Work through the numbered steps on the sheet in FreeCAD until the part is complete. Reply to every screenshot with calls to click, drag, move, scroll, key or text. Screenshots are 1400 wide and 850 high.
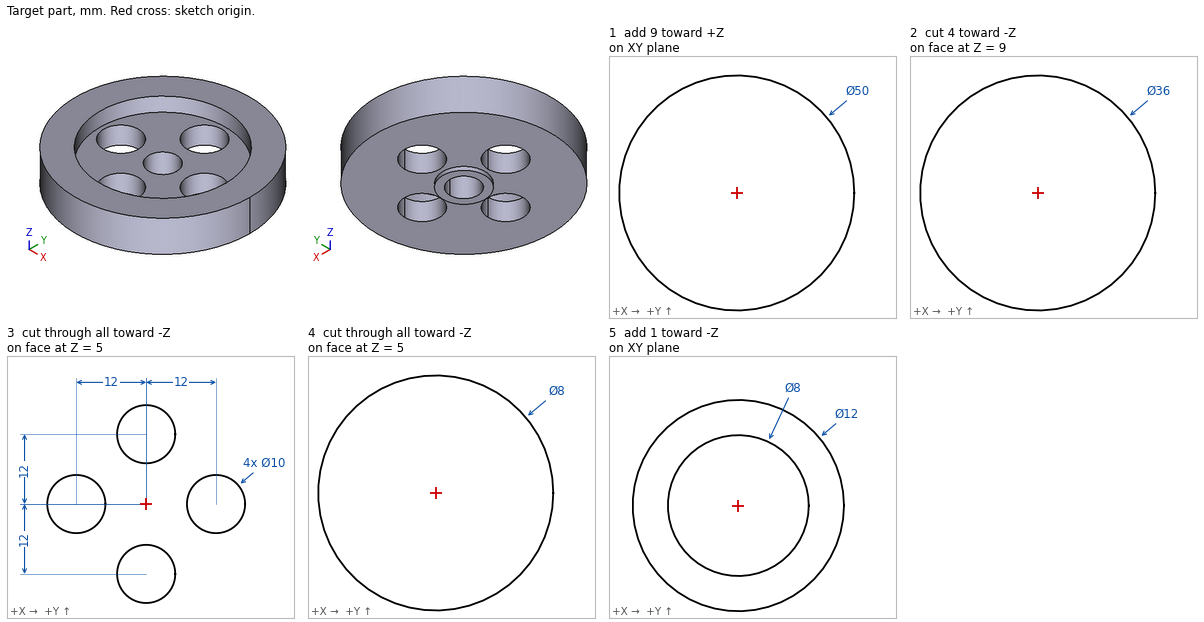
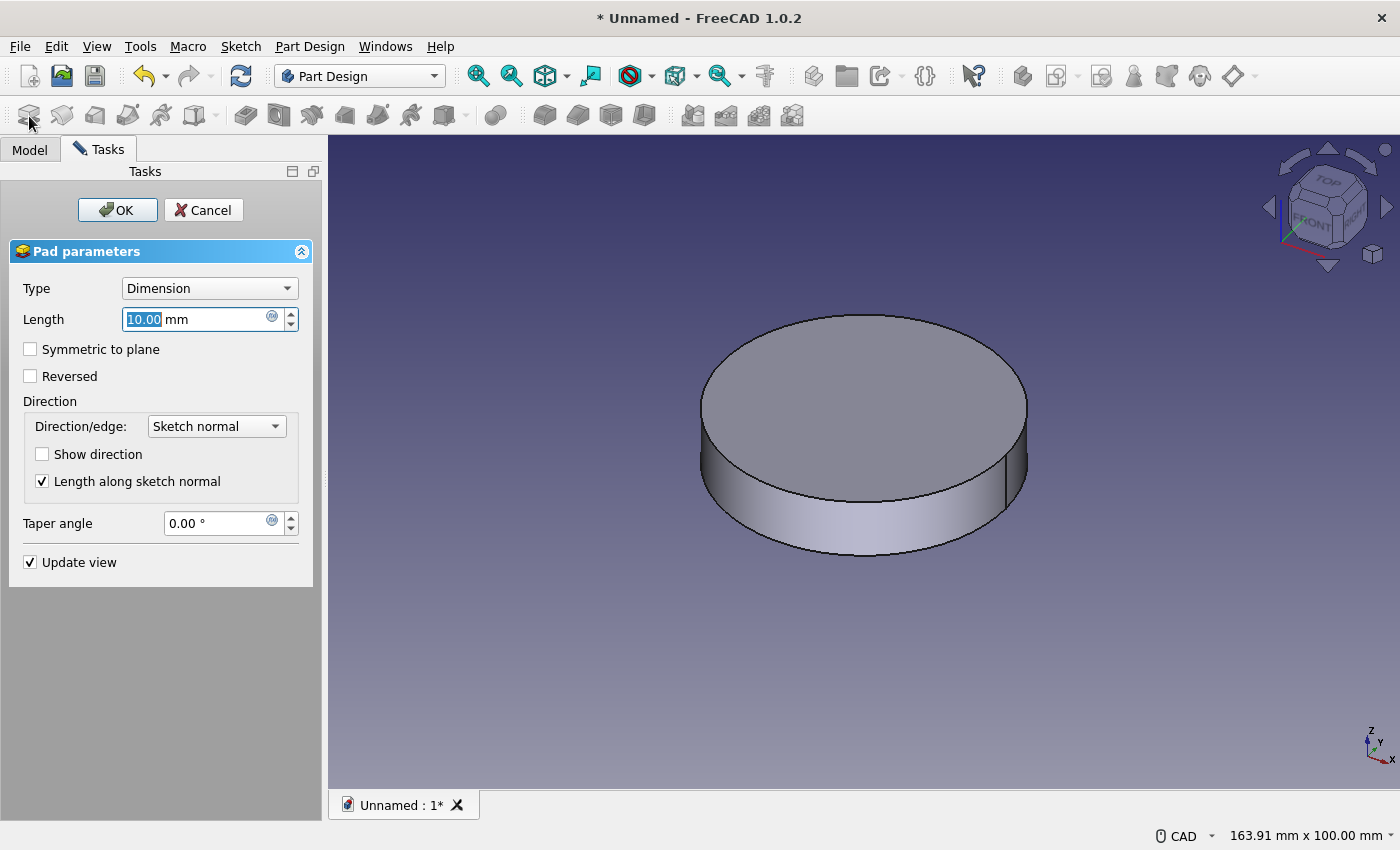
text(9)
key(Tab)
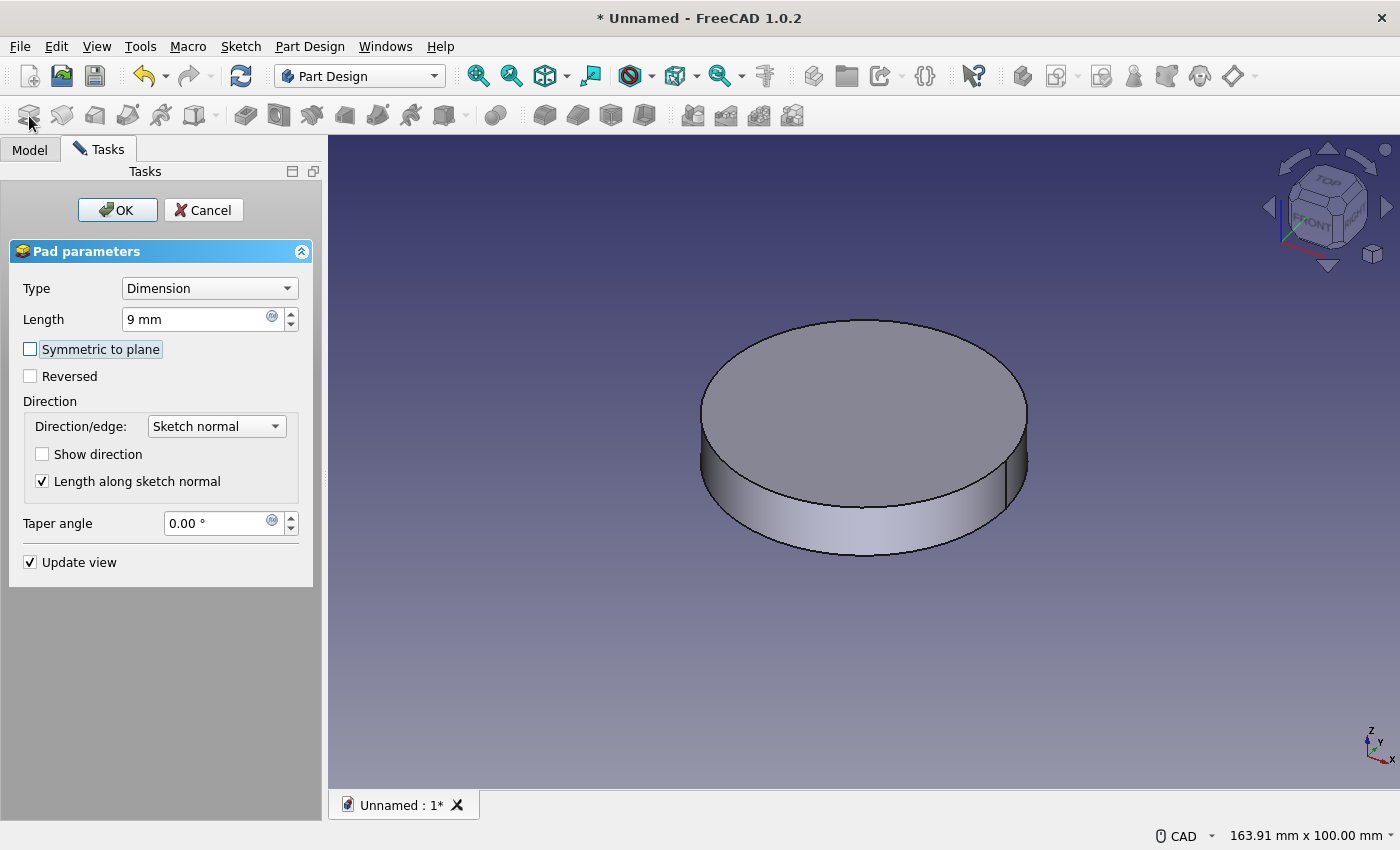
click(118, 210)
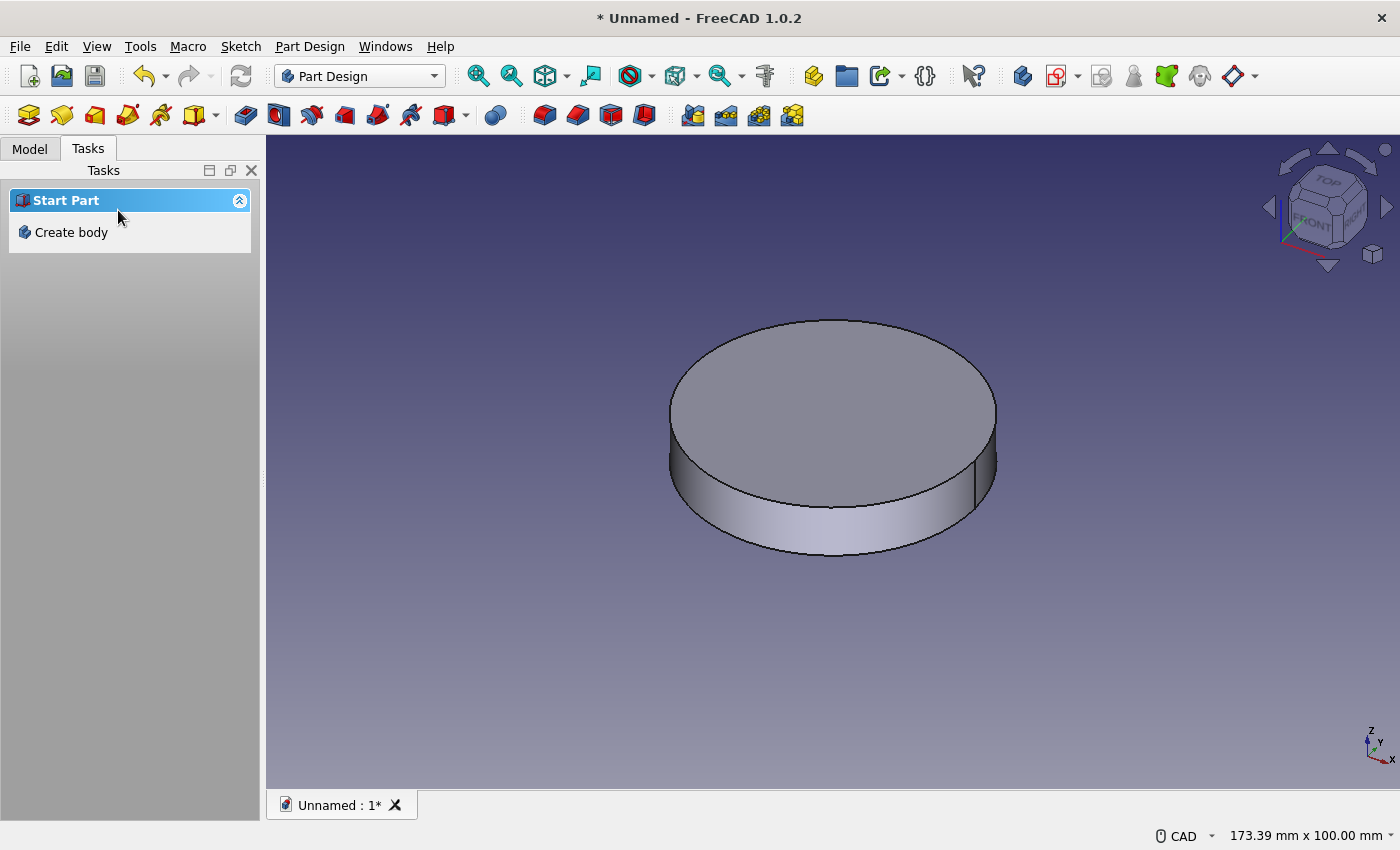
click(833, 413)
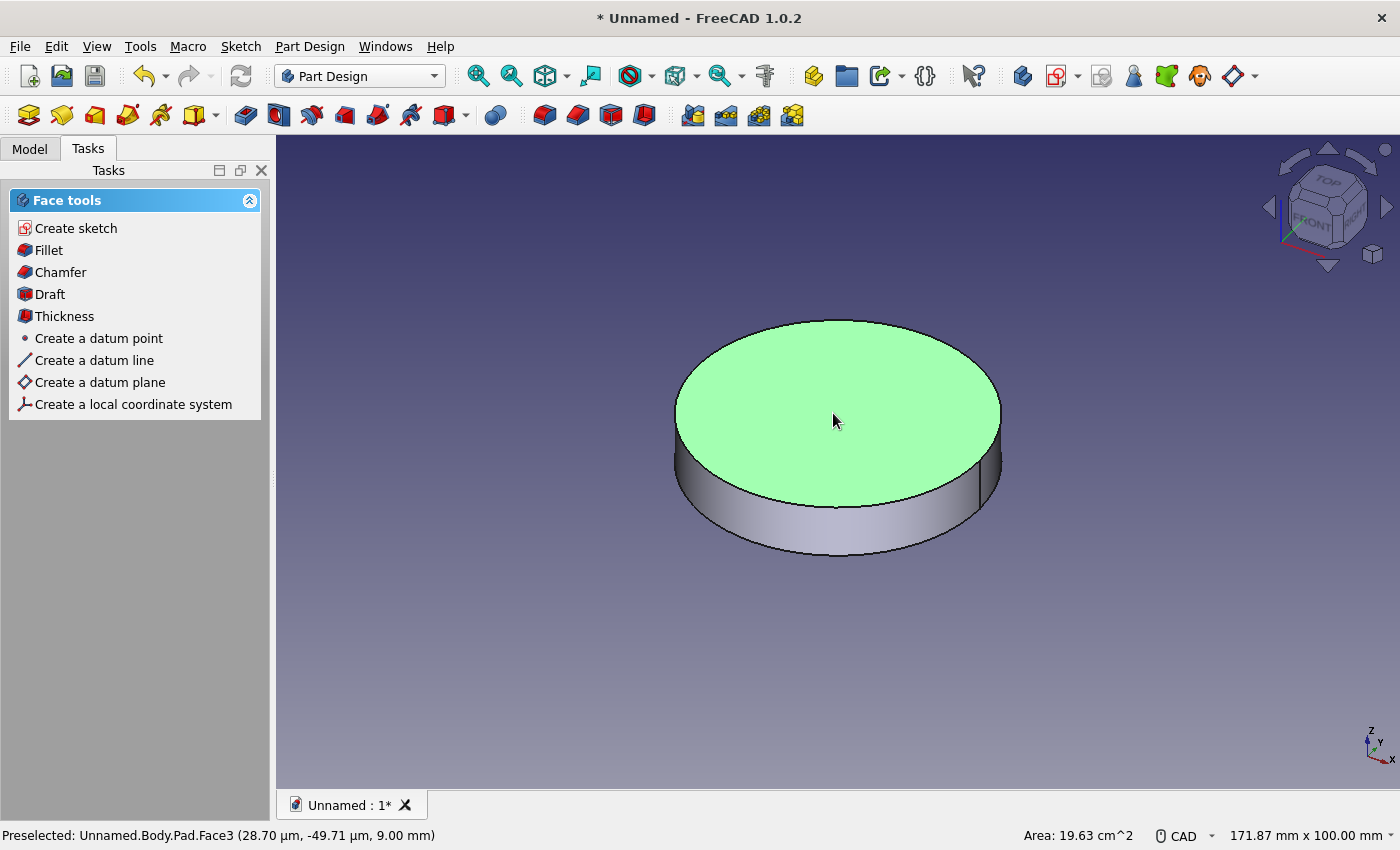
click(1056, 76)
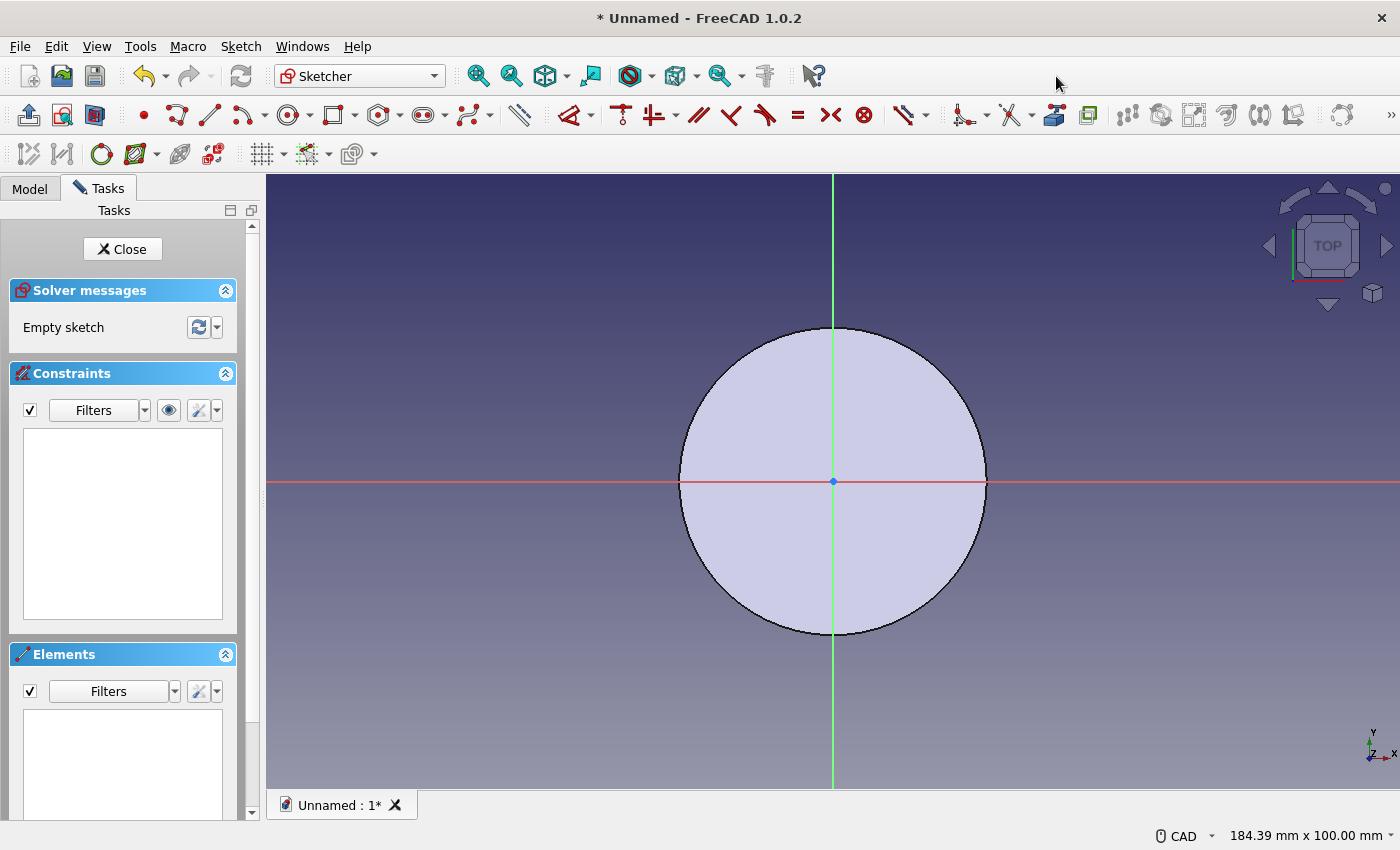
scroll(916, 481, up, 3)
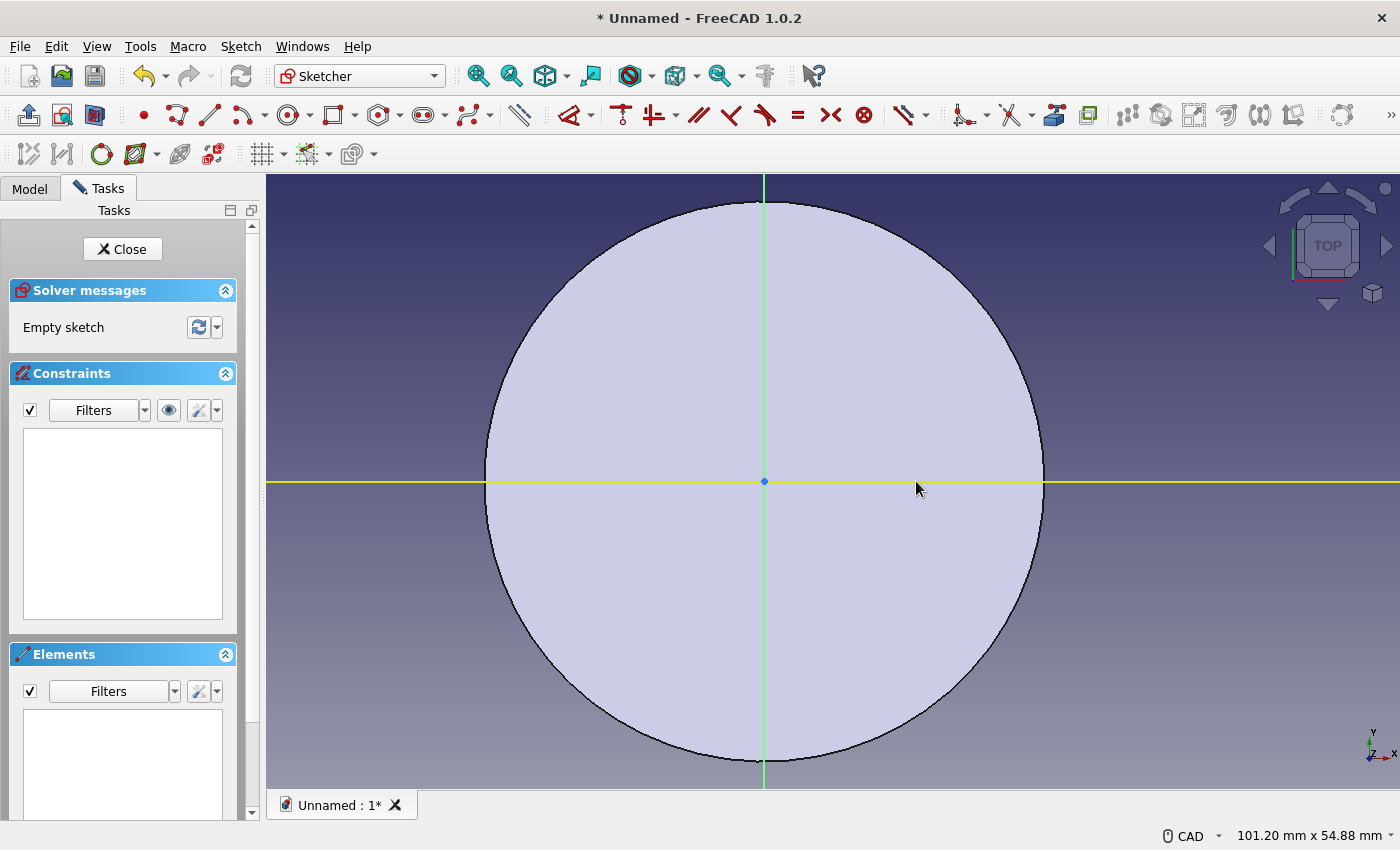
click(288, 116)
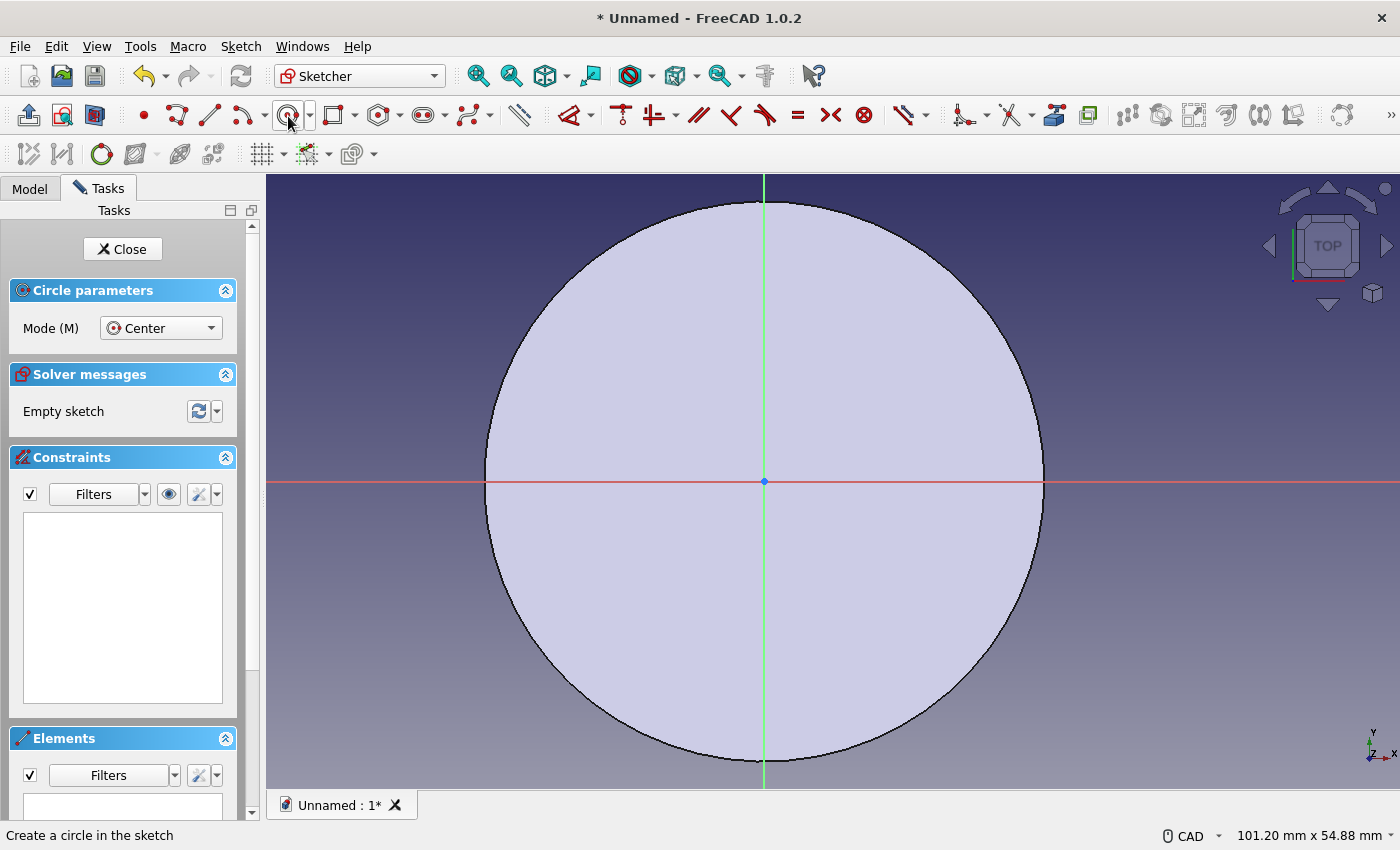
click(764, 482)
move(907, 339)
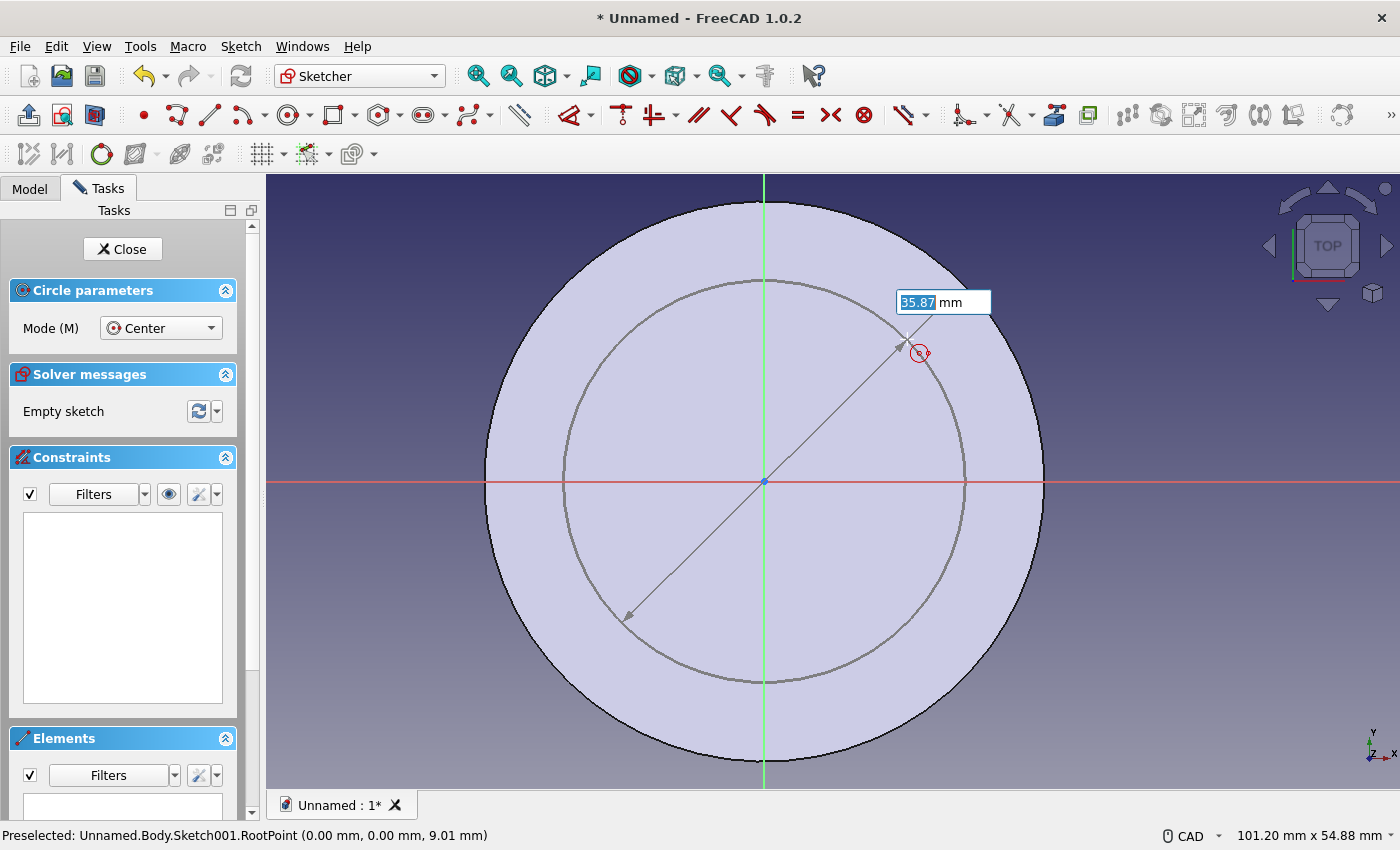
text(36)
key(Return)
key(Escape)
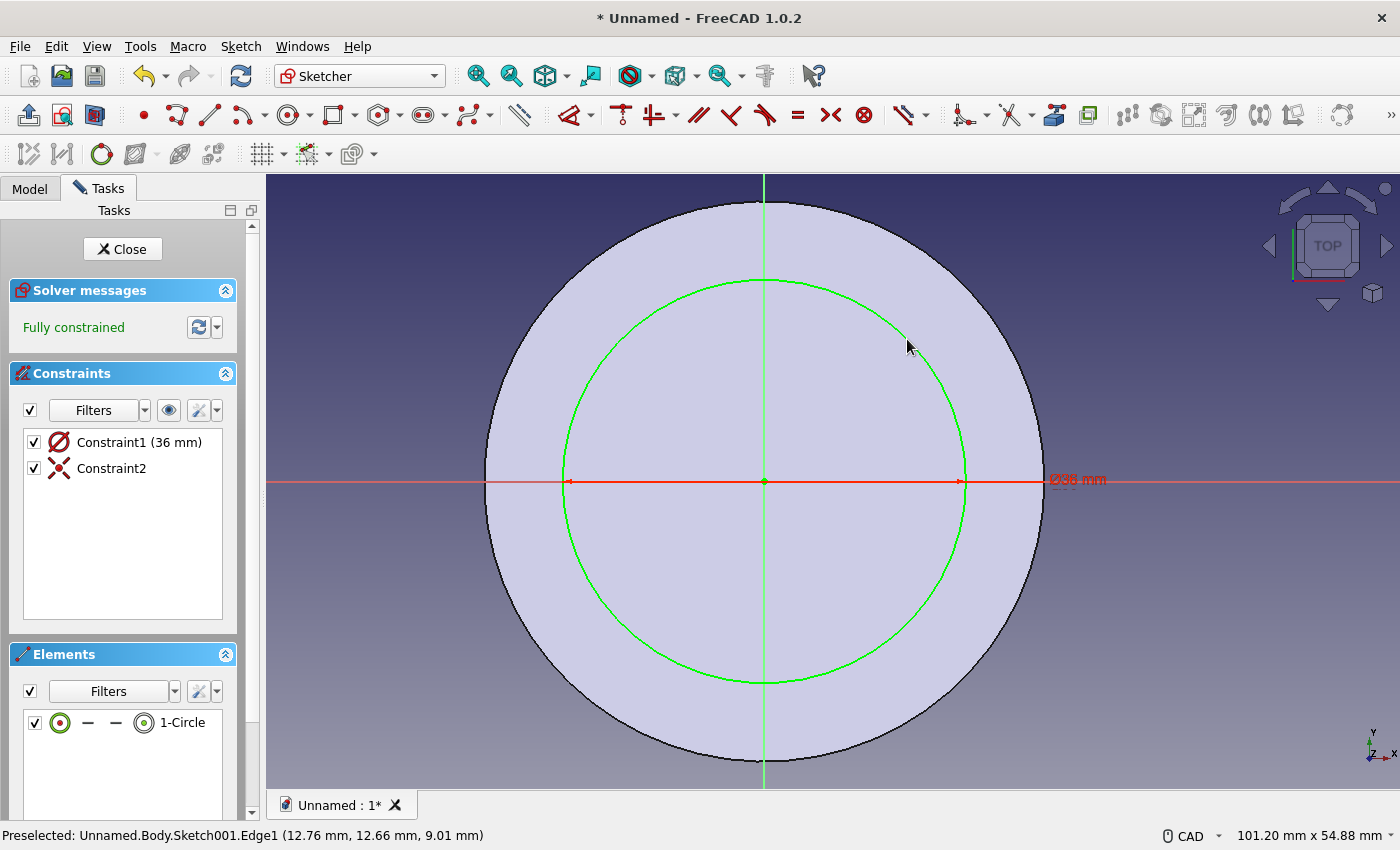
click(123, 249)